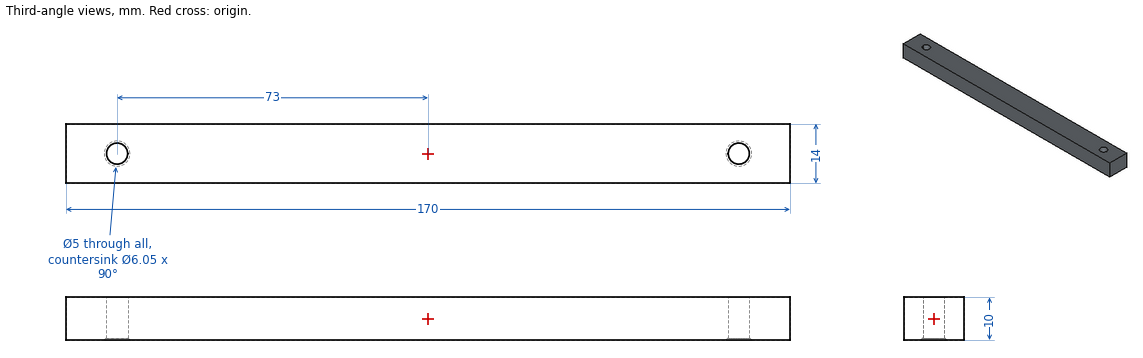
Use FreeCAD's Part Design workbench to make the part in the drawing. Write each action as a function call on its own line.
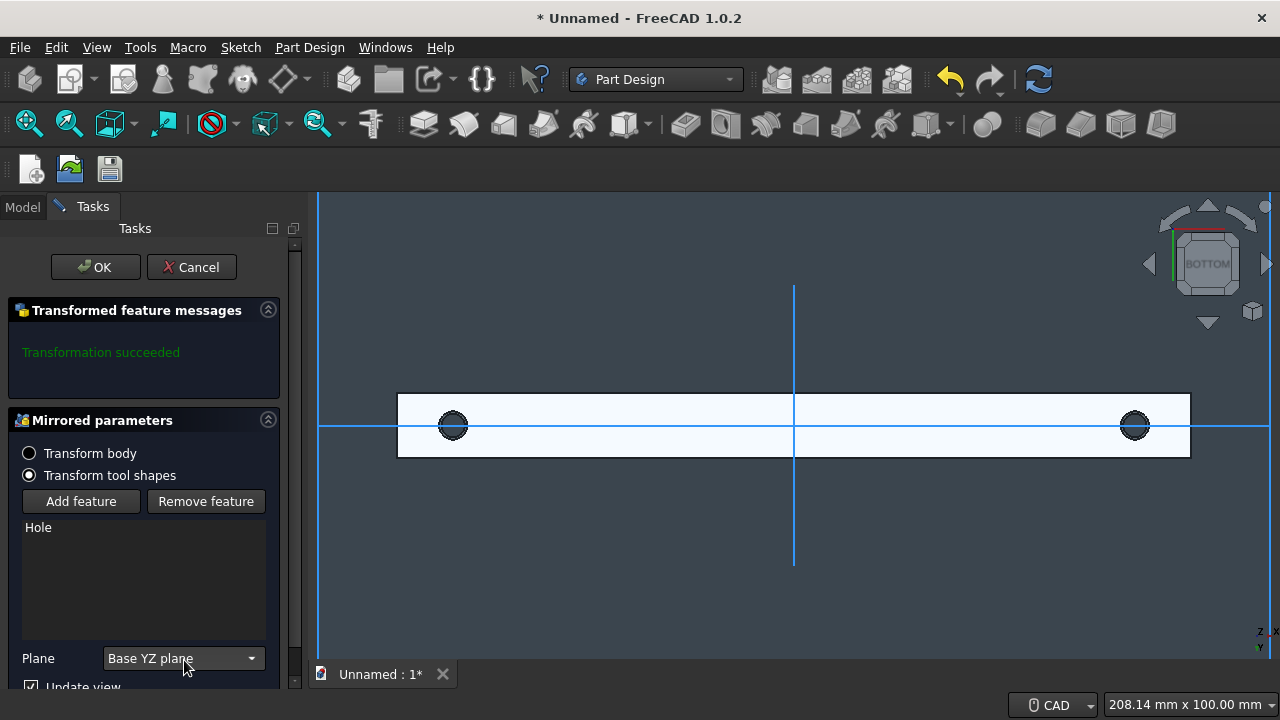
click(96, 267)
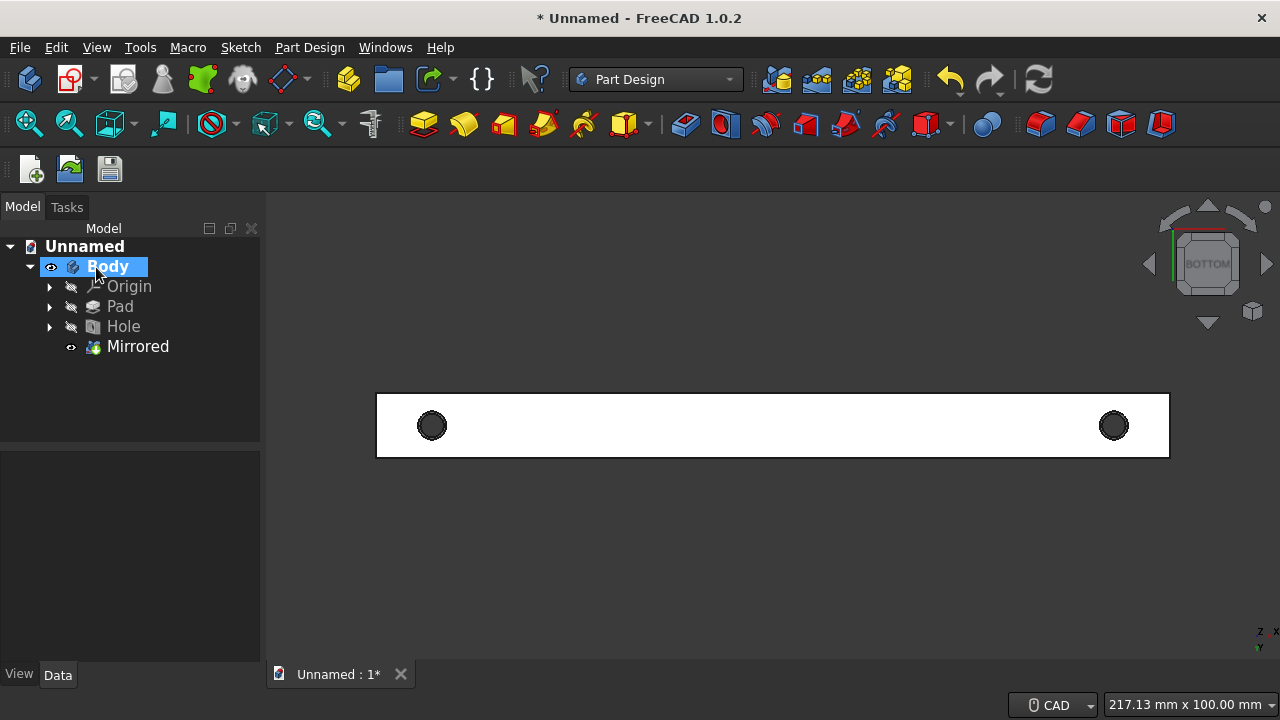
key(0)